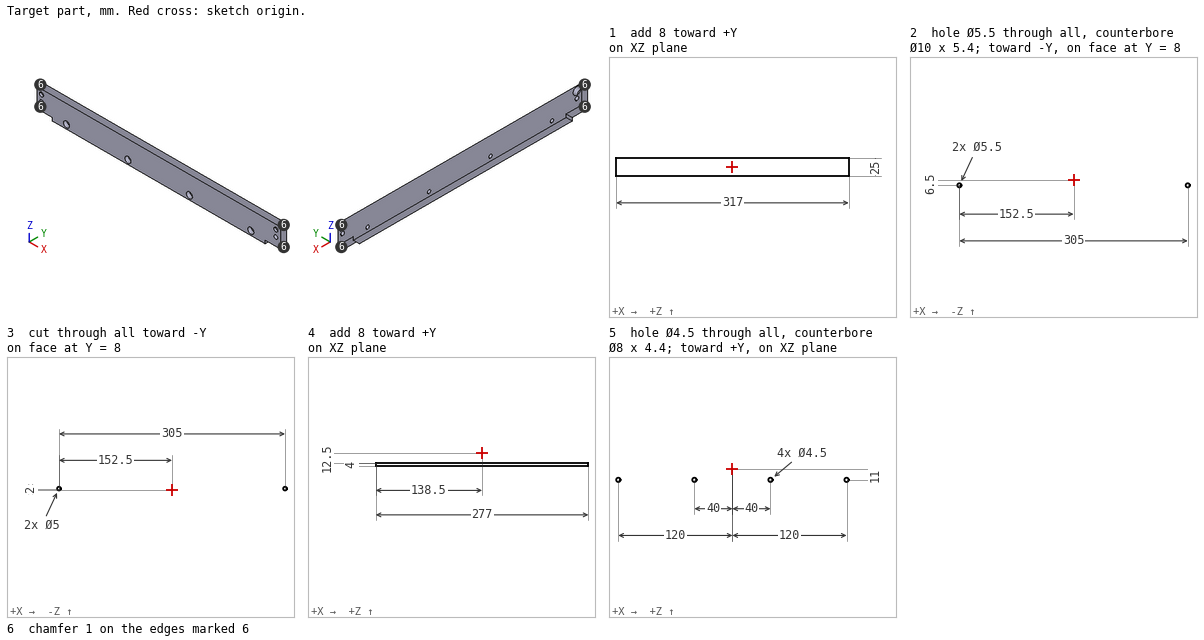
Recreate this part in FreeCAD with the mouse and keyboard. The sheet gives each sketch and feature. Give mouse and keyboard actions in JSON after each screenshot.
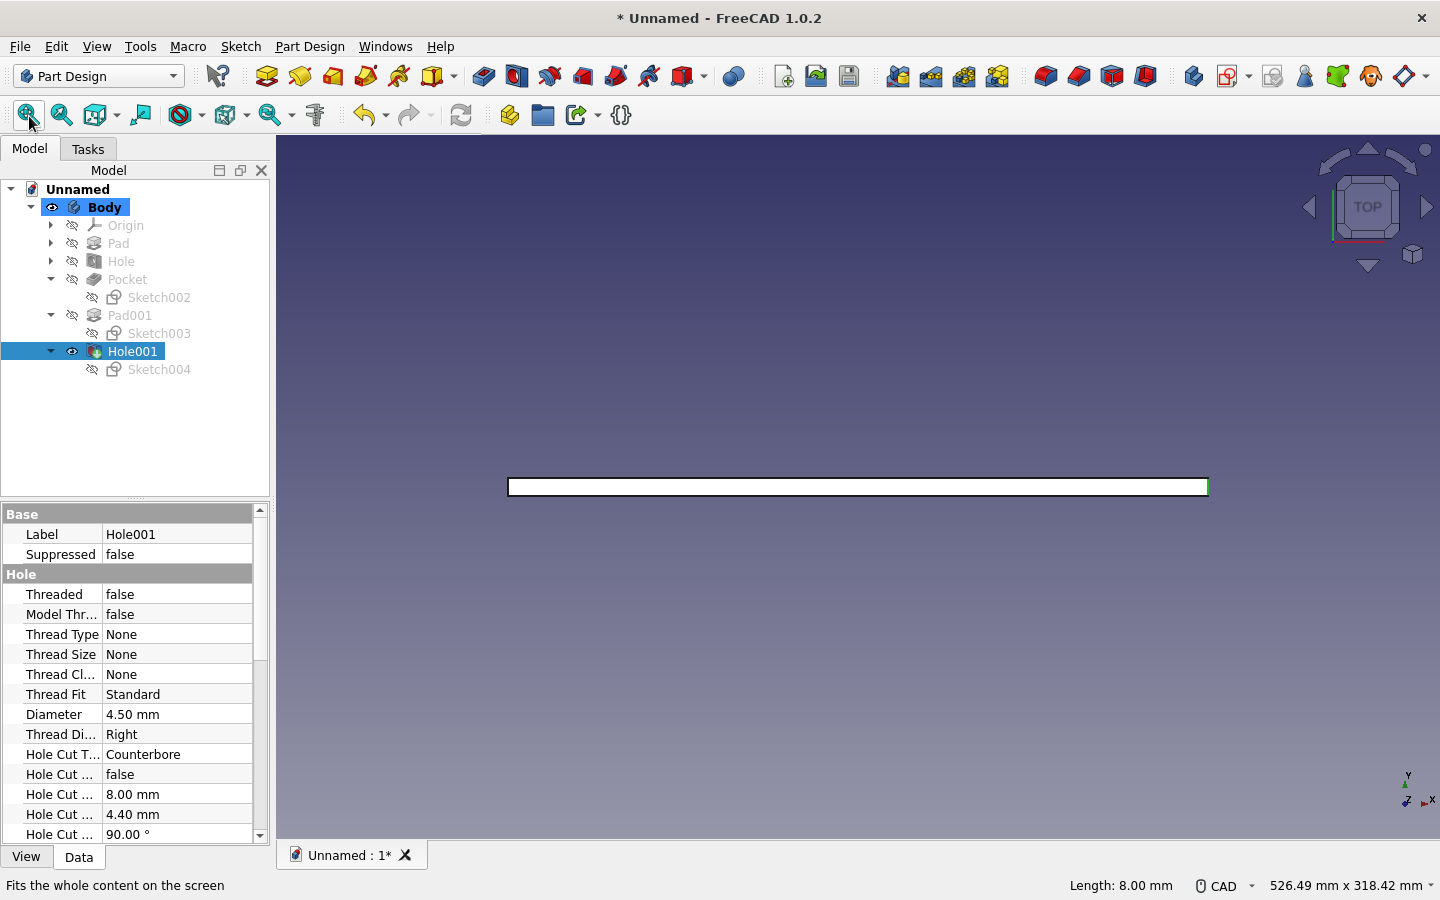
{"action": "left_click", "coordinate": [508, 486], "text": "ctrl"}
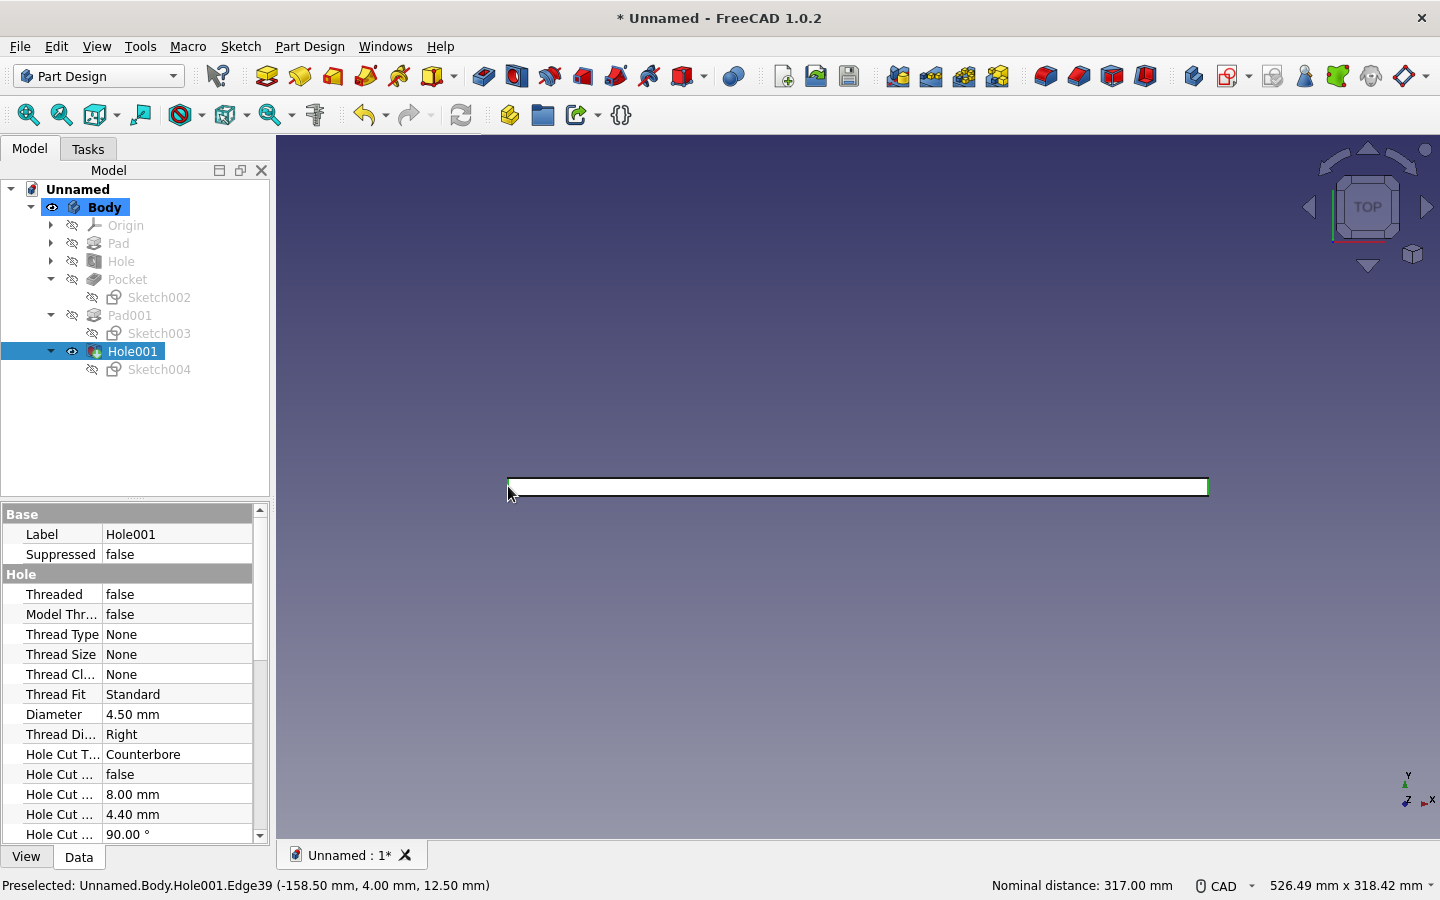
{"action": "scroll", "coordinate": [508, 486], "scroll_direction": "up", "scroll_amount": 5}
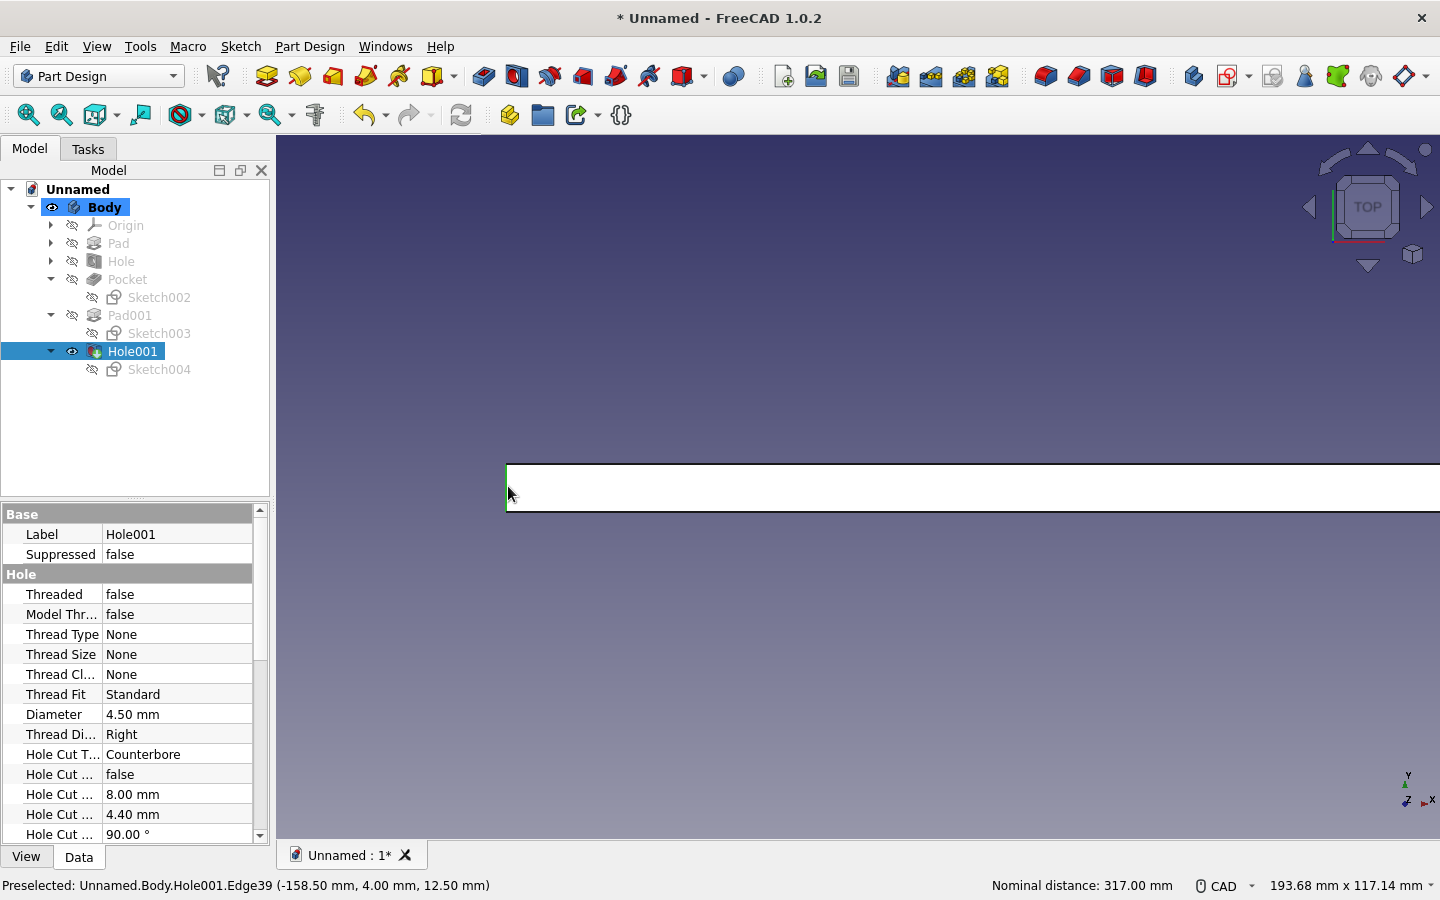
{"action": "left_click", "coordinate": [29, 116]}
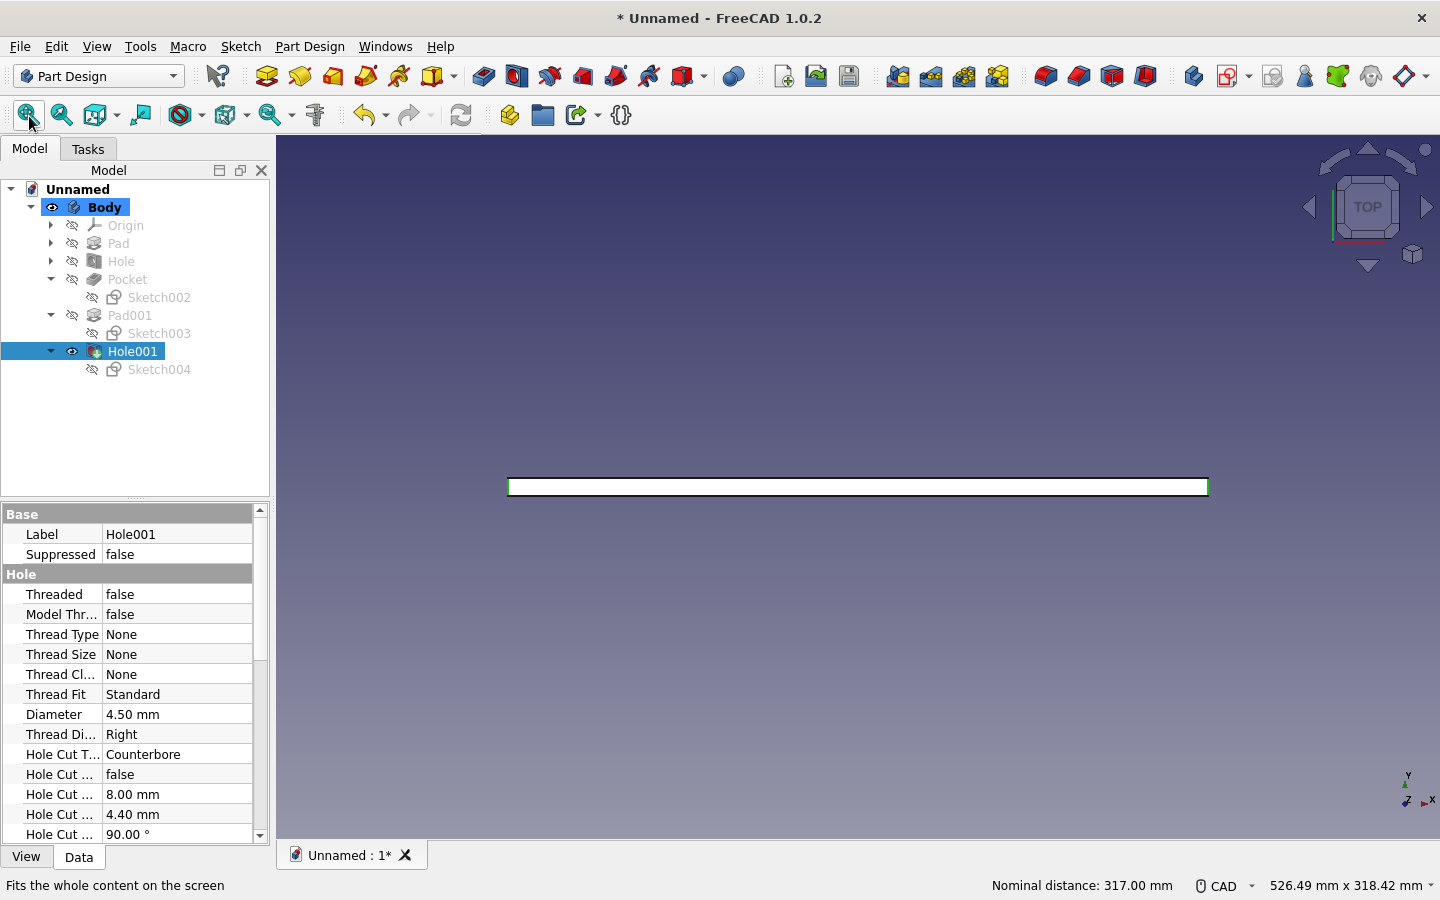
{"action": "key", "text": "1"}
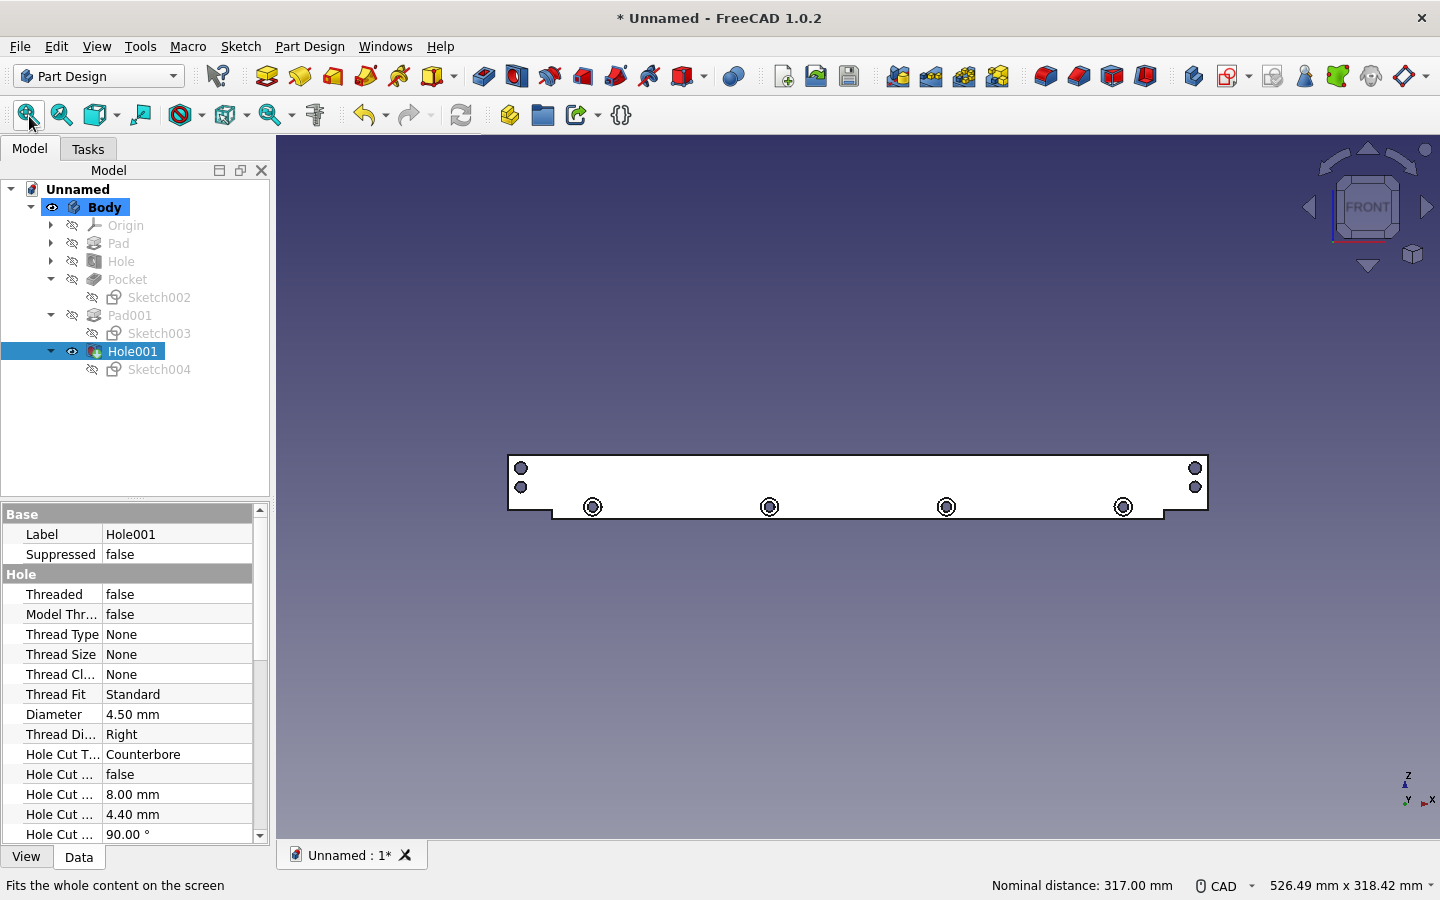
{"action": "scroll", "coordinate": [508, 509], "scroll_direction": "up", "scroll_amount": 5}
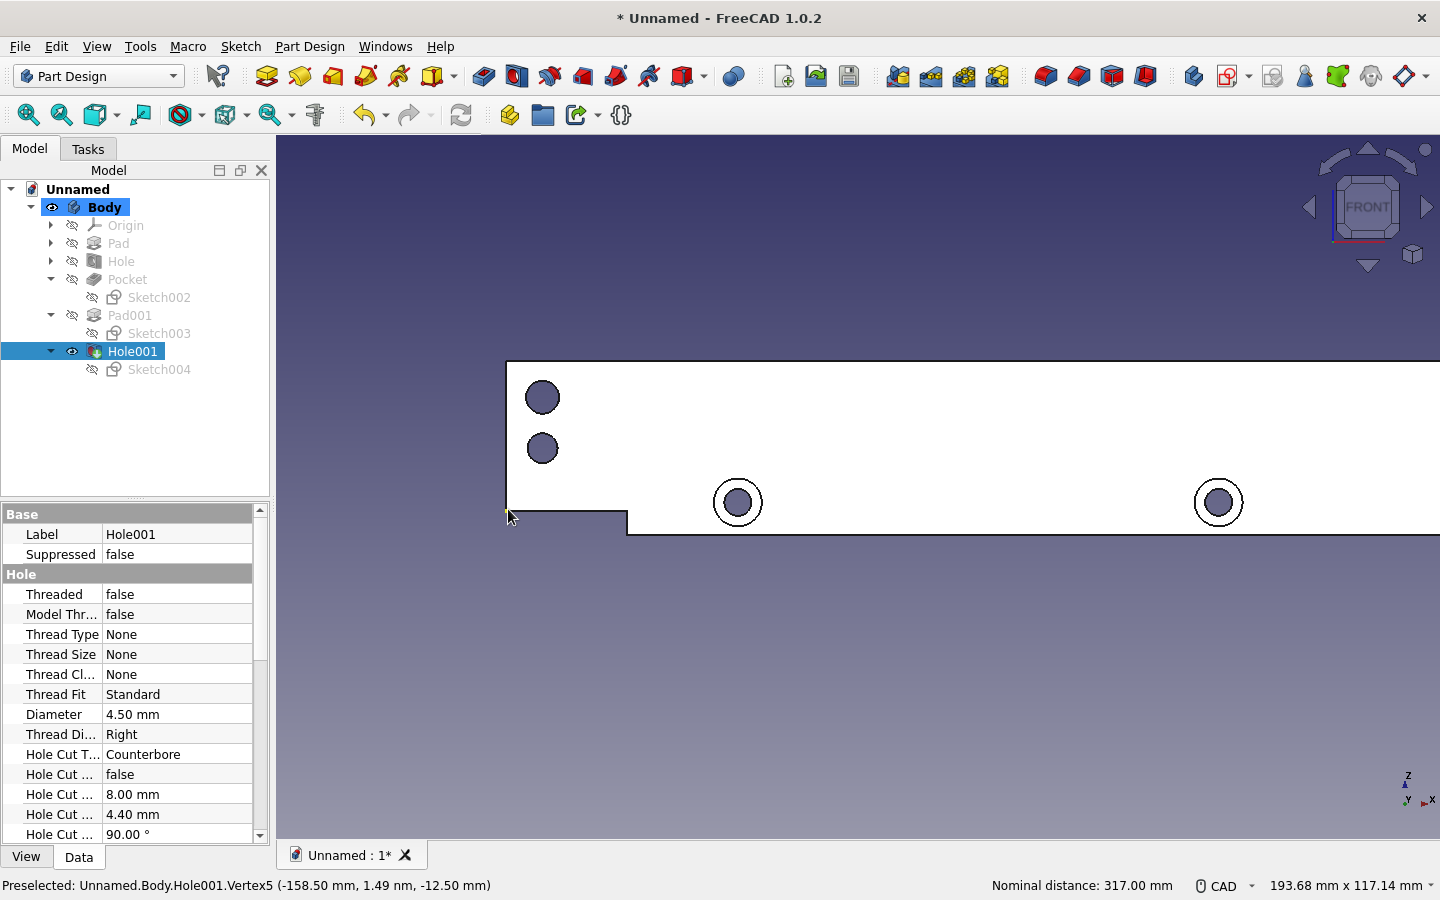
{"action": "left_click", "coordinate": [29, 116]}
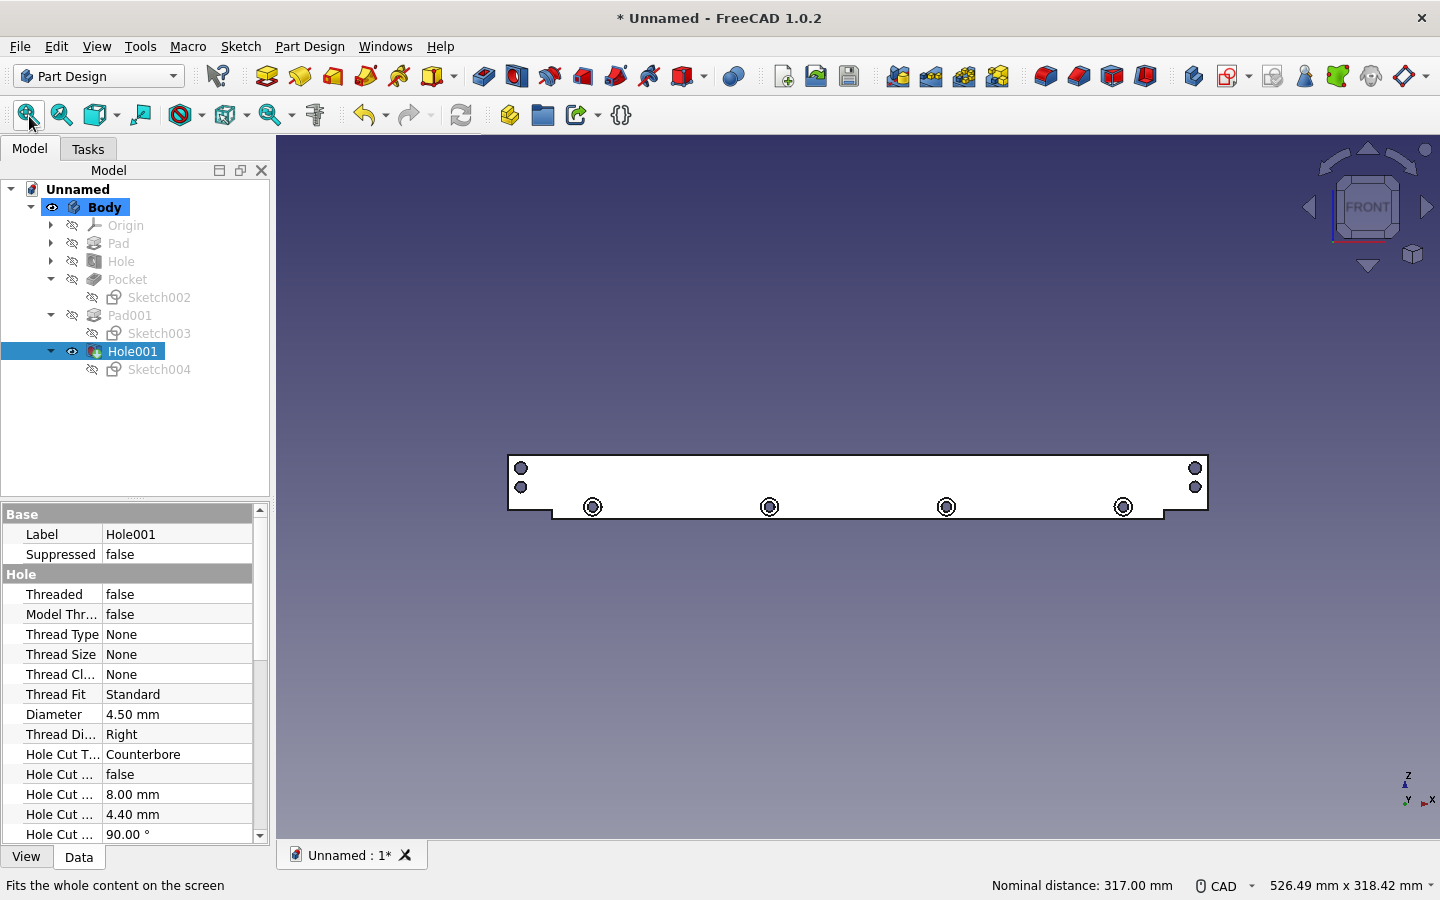
{"action": "key", "text": "3"}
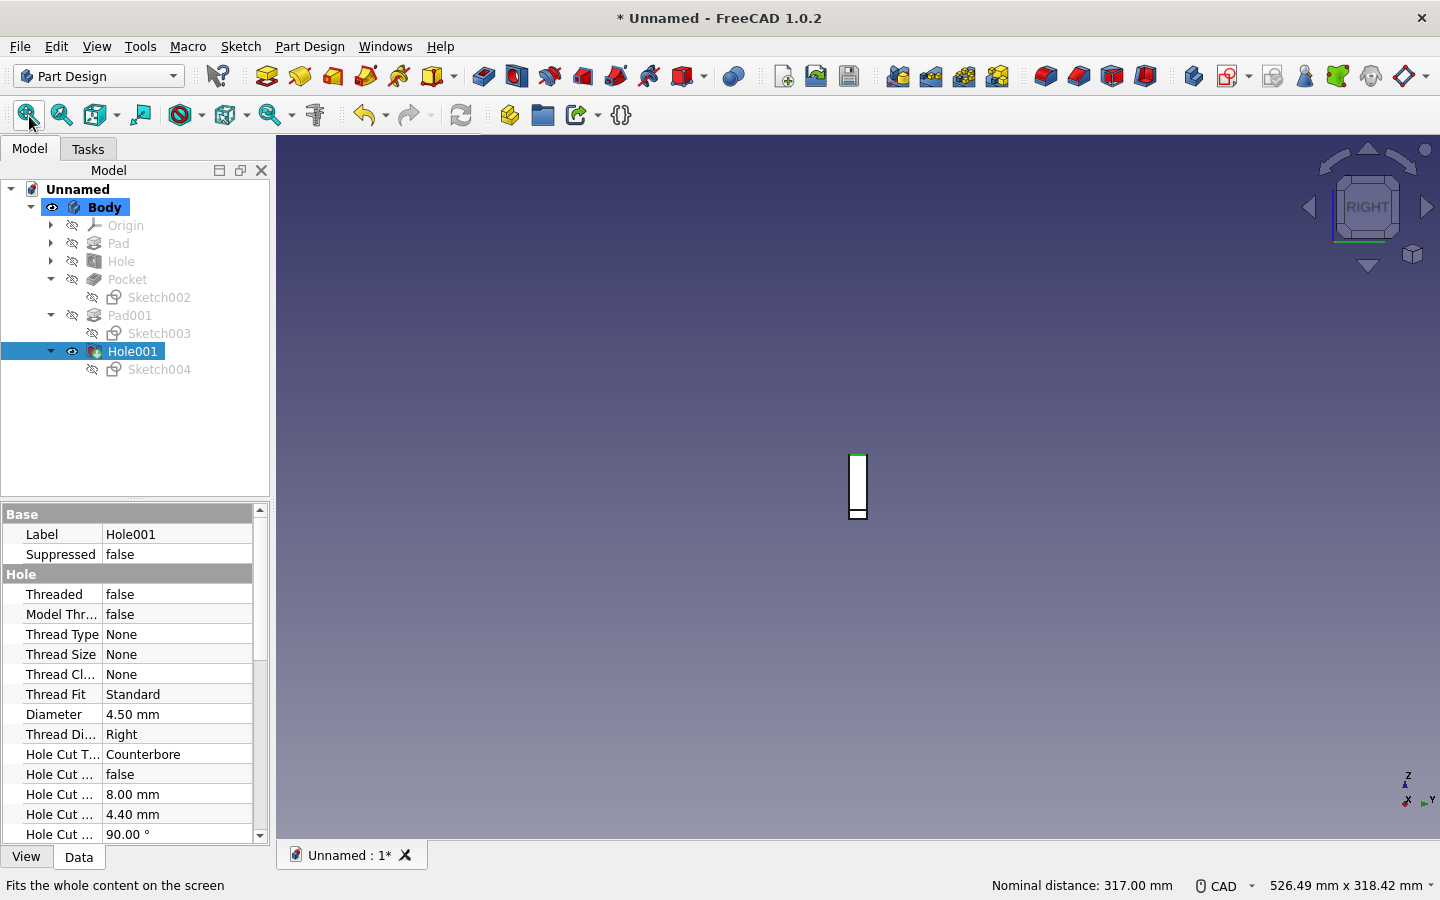
{"action": "left_click", "coordinate": [29, 116]}